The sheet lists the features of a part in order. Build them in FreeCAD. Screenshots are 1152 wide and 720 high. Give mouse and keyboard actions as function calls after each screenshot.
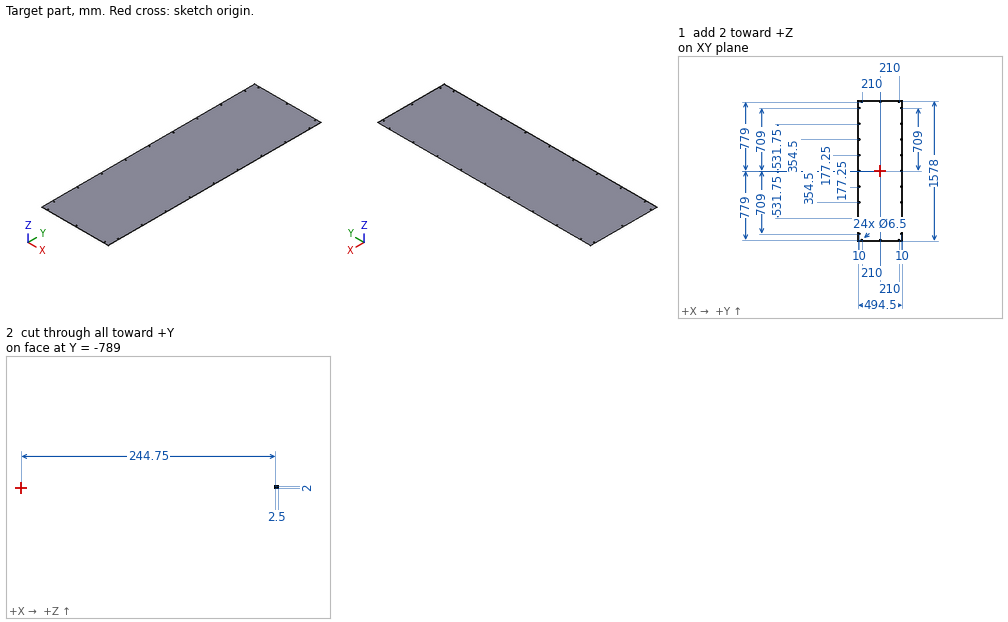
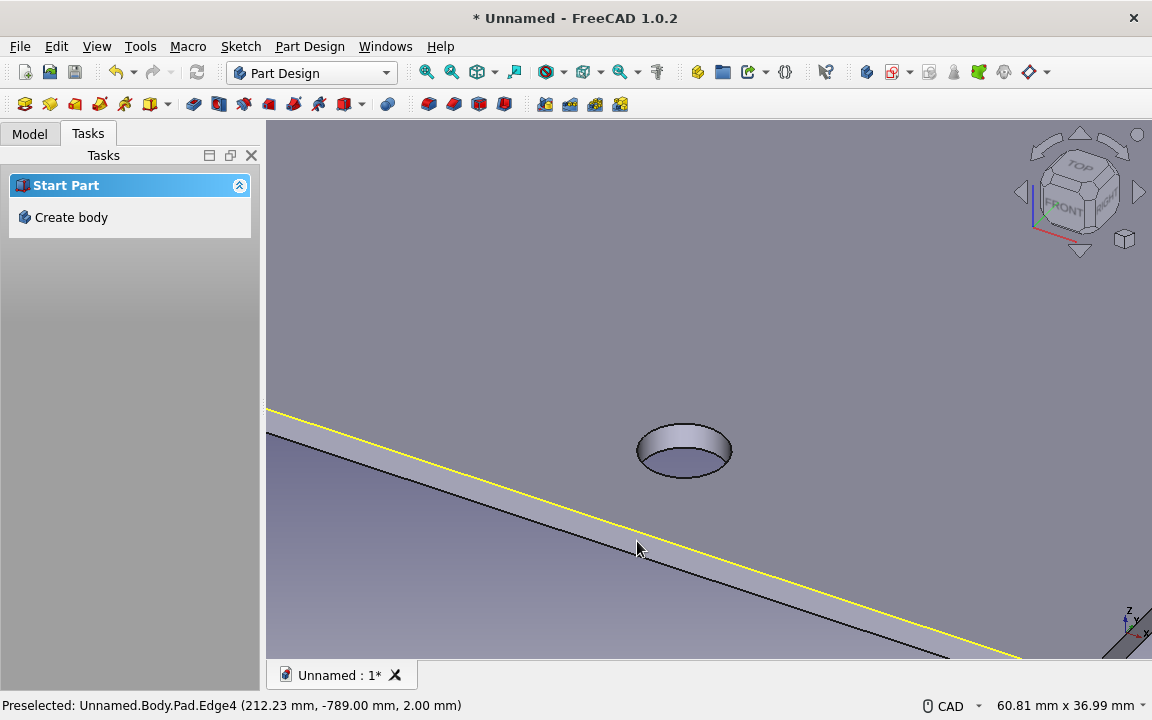
click(636, 542)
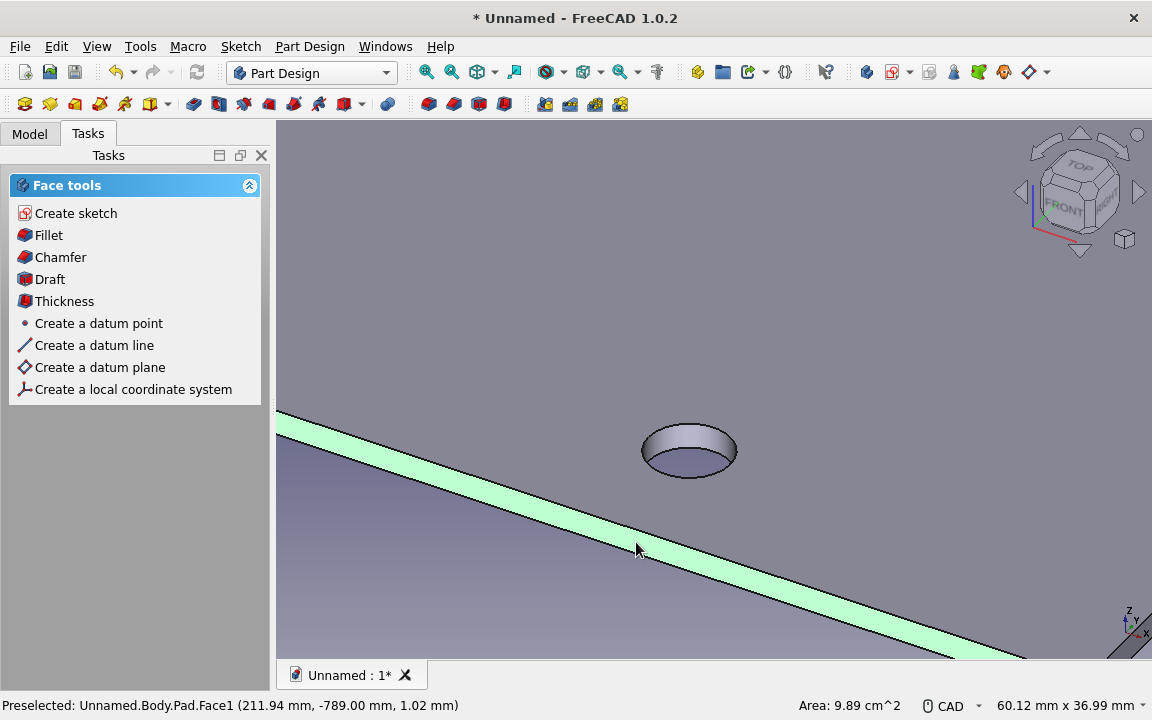
click(892, 72)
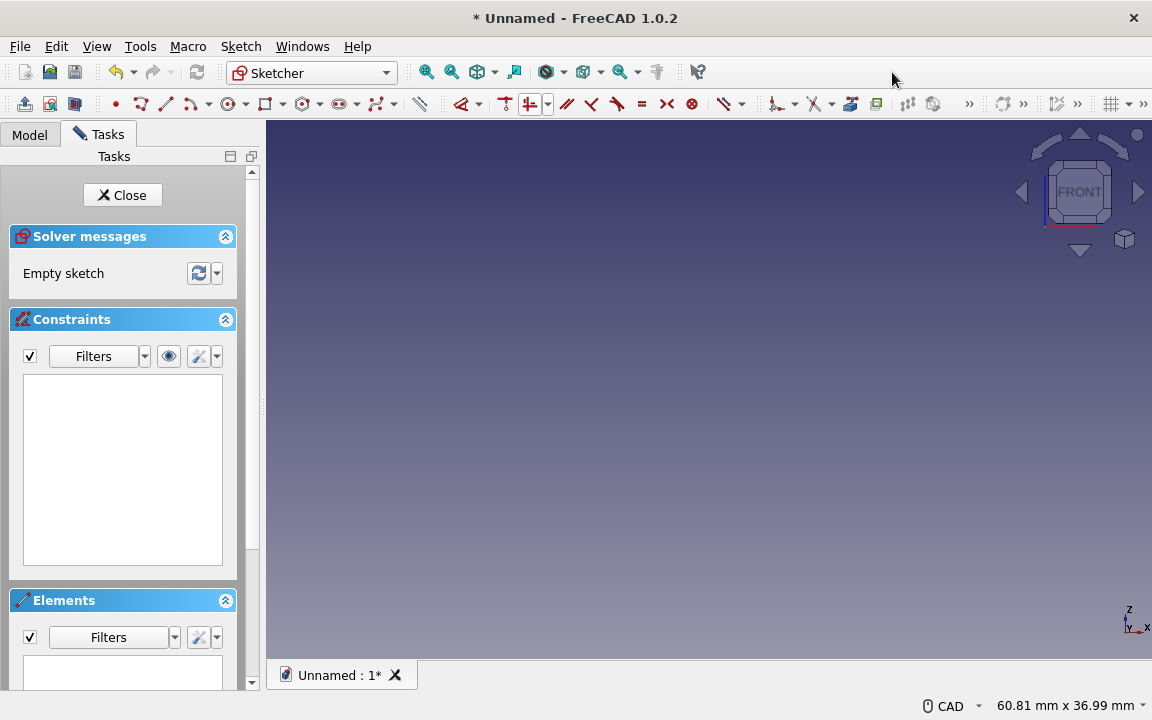
scroll(640, 390, down, 5)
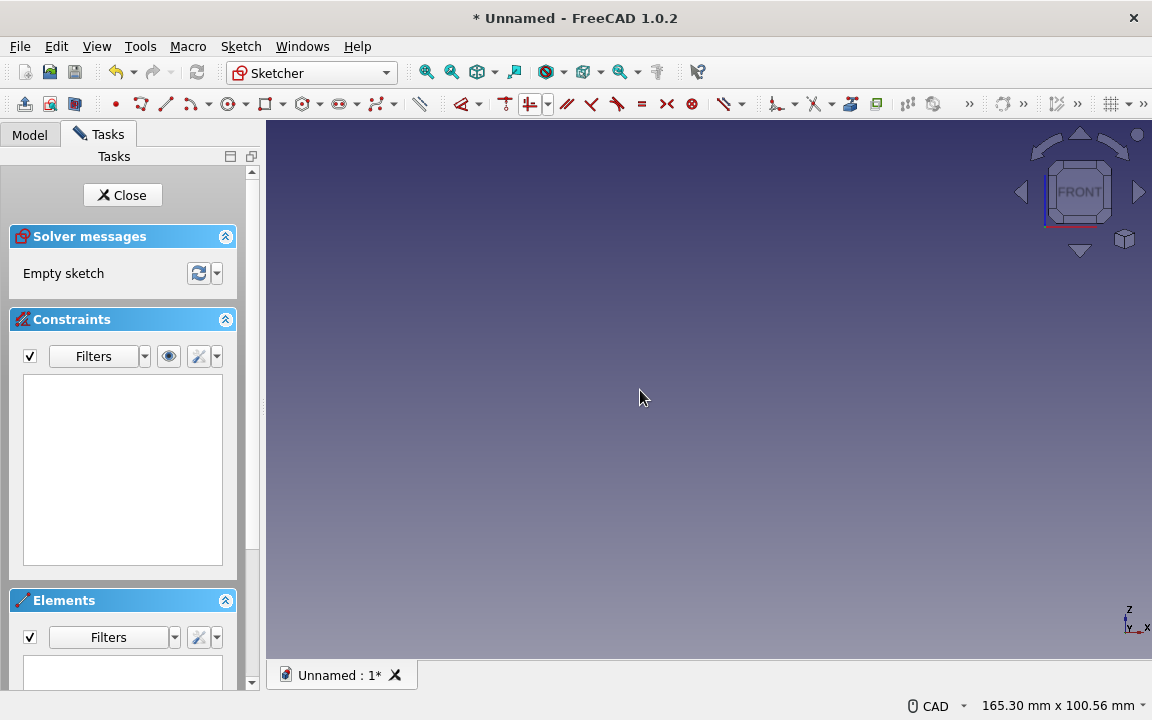
scroll(640, 390, down, 5)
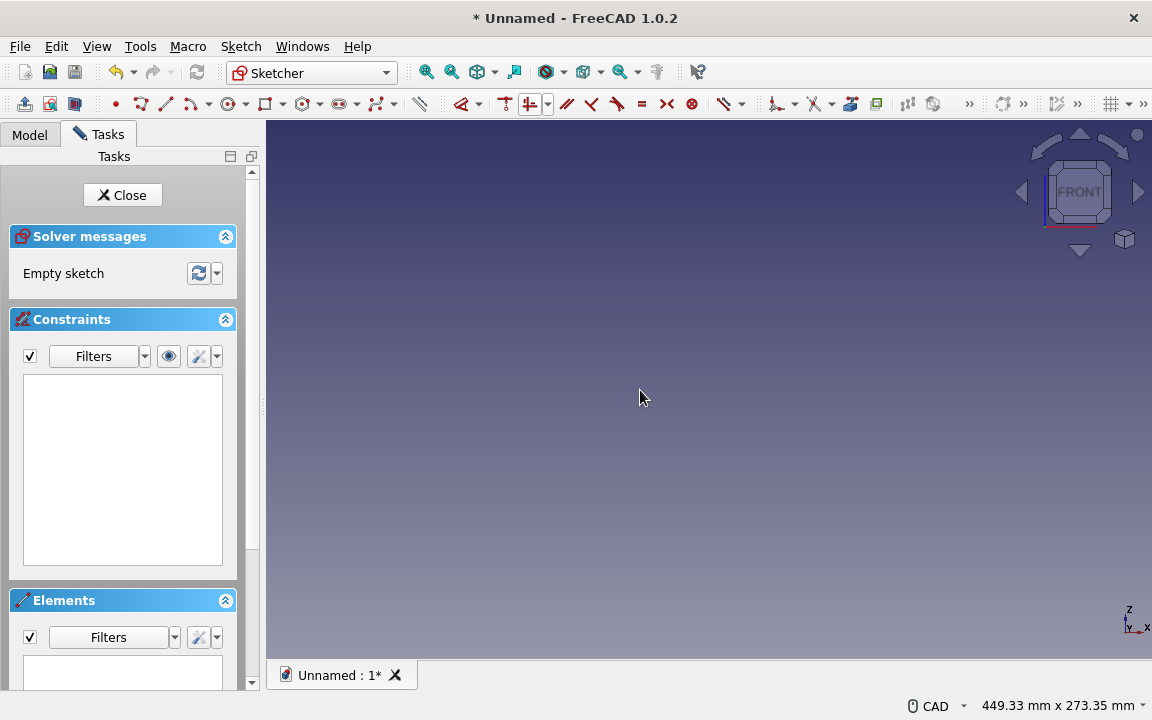
scroll(640, 390, down, 5)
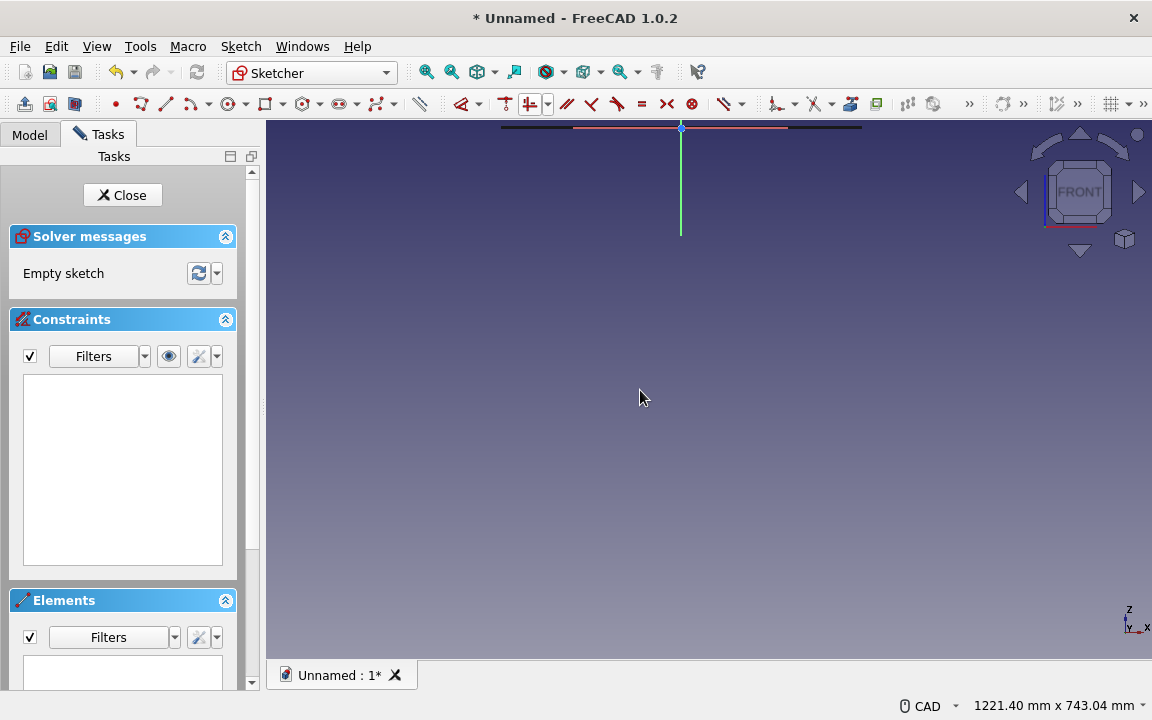
scroll(640, 390, down, 5)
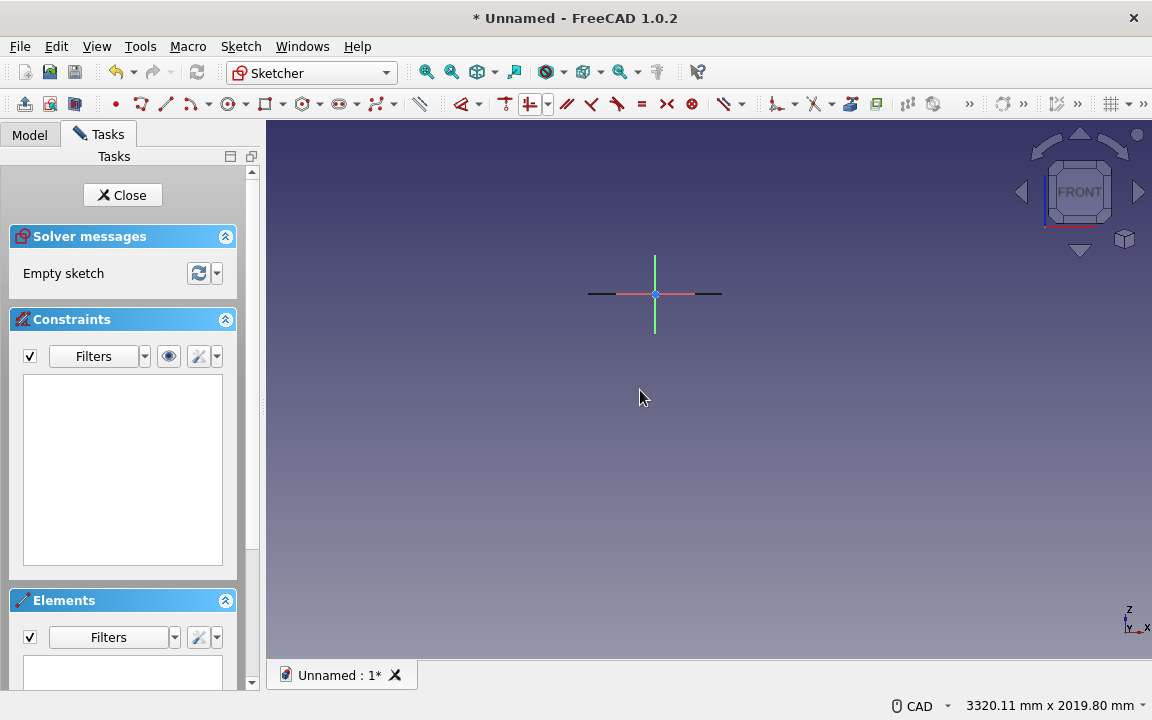
scroll(725, 289, up, 15)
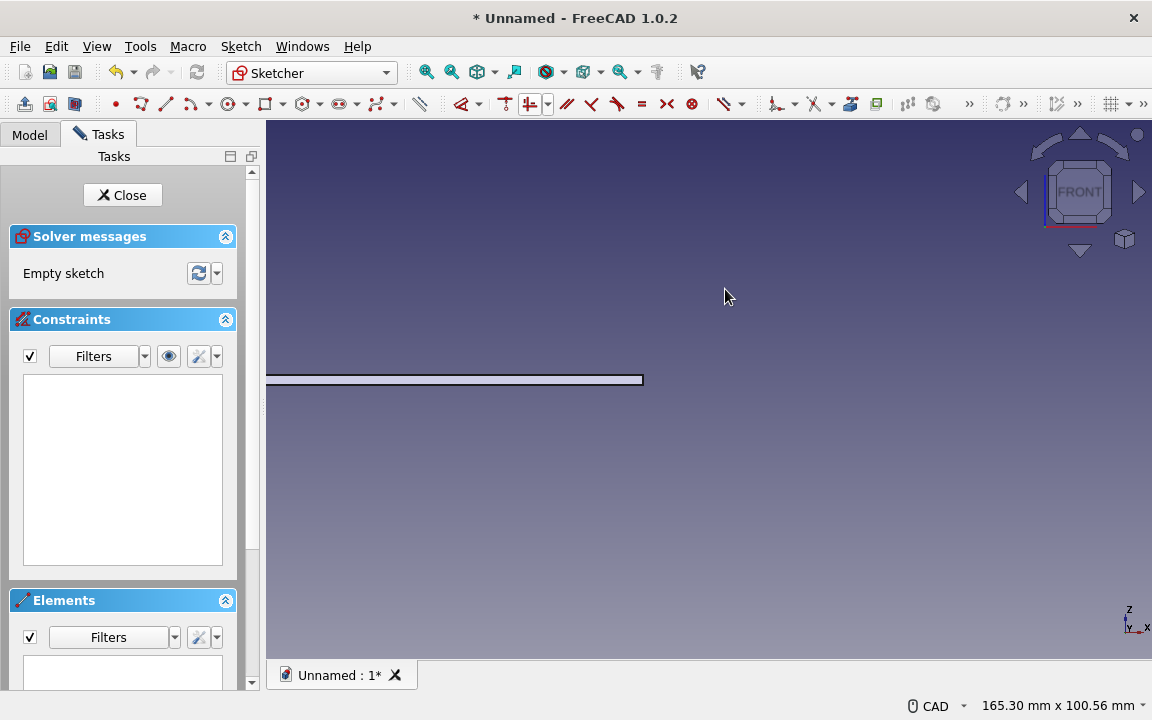
click(264, 104)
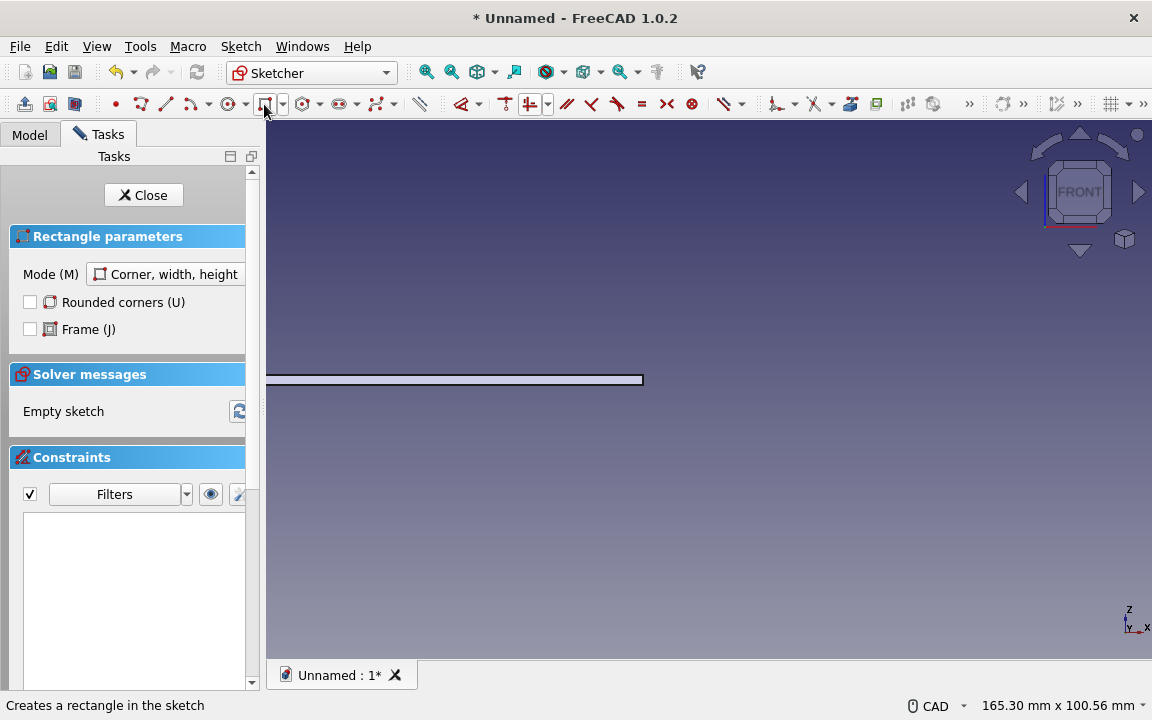
scroll(630, 375, up, 2)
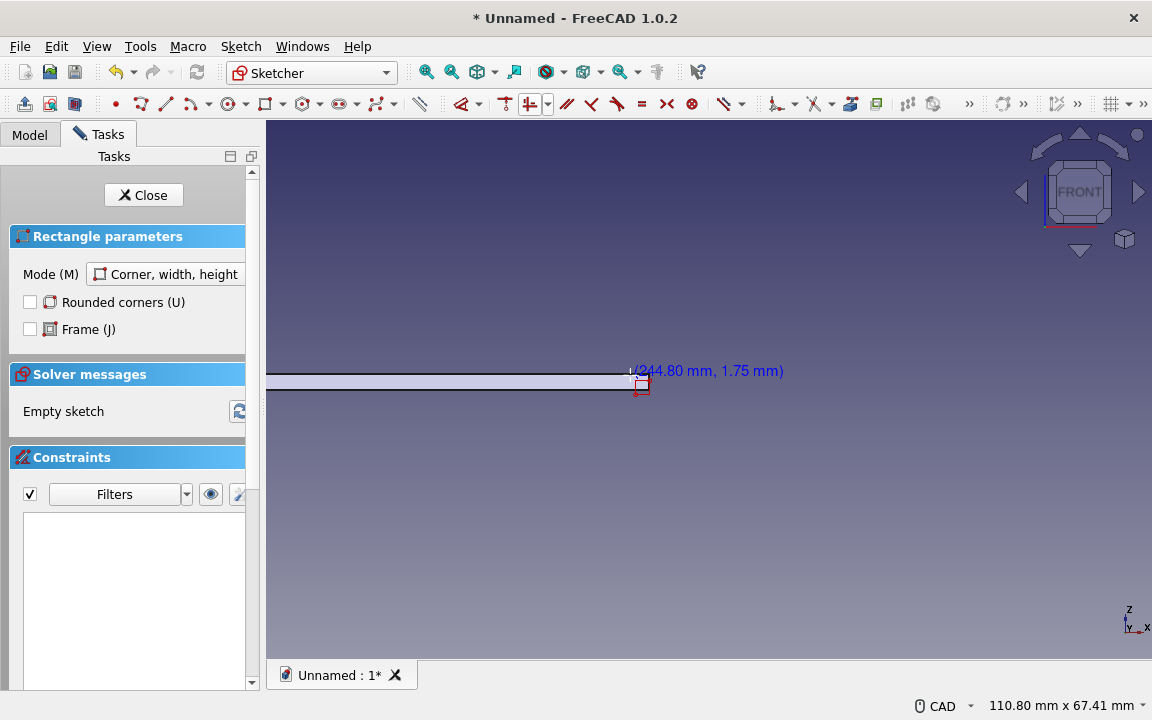
click(629, 374)
click(649, 390)
key(Escape)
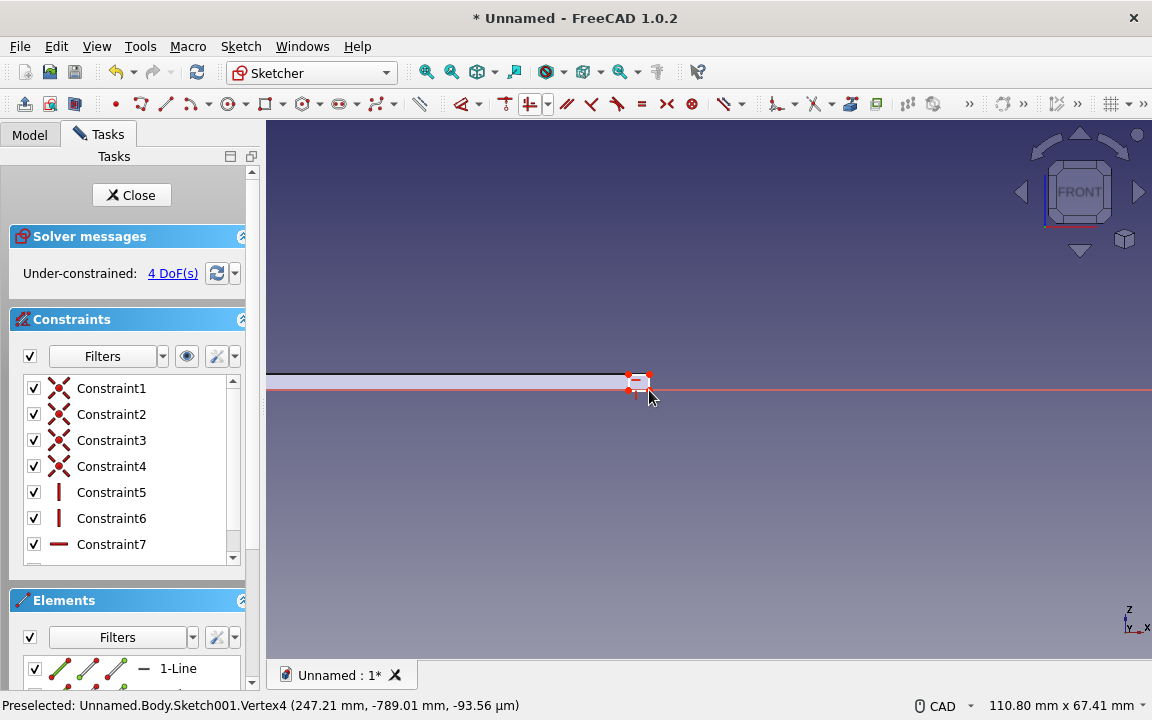
click(629, 391)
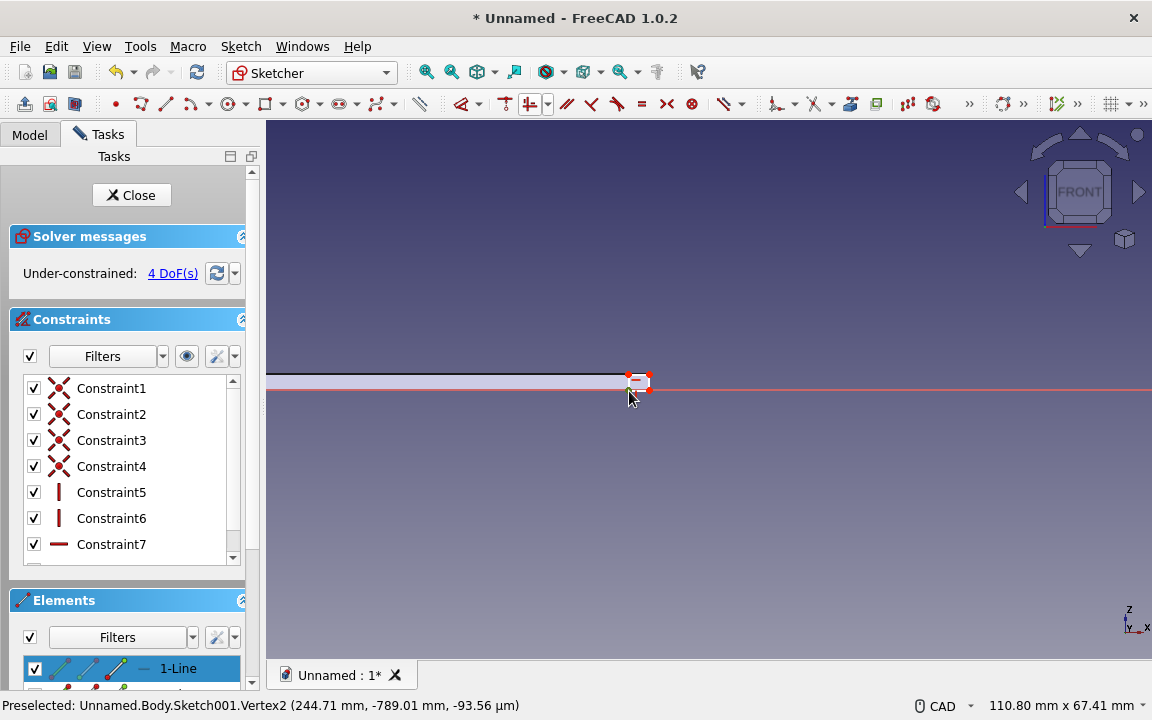
click(343, 390)